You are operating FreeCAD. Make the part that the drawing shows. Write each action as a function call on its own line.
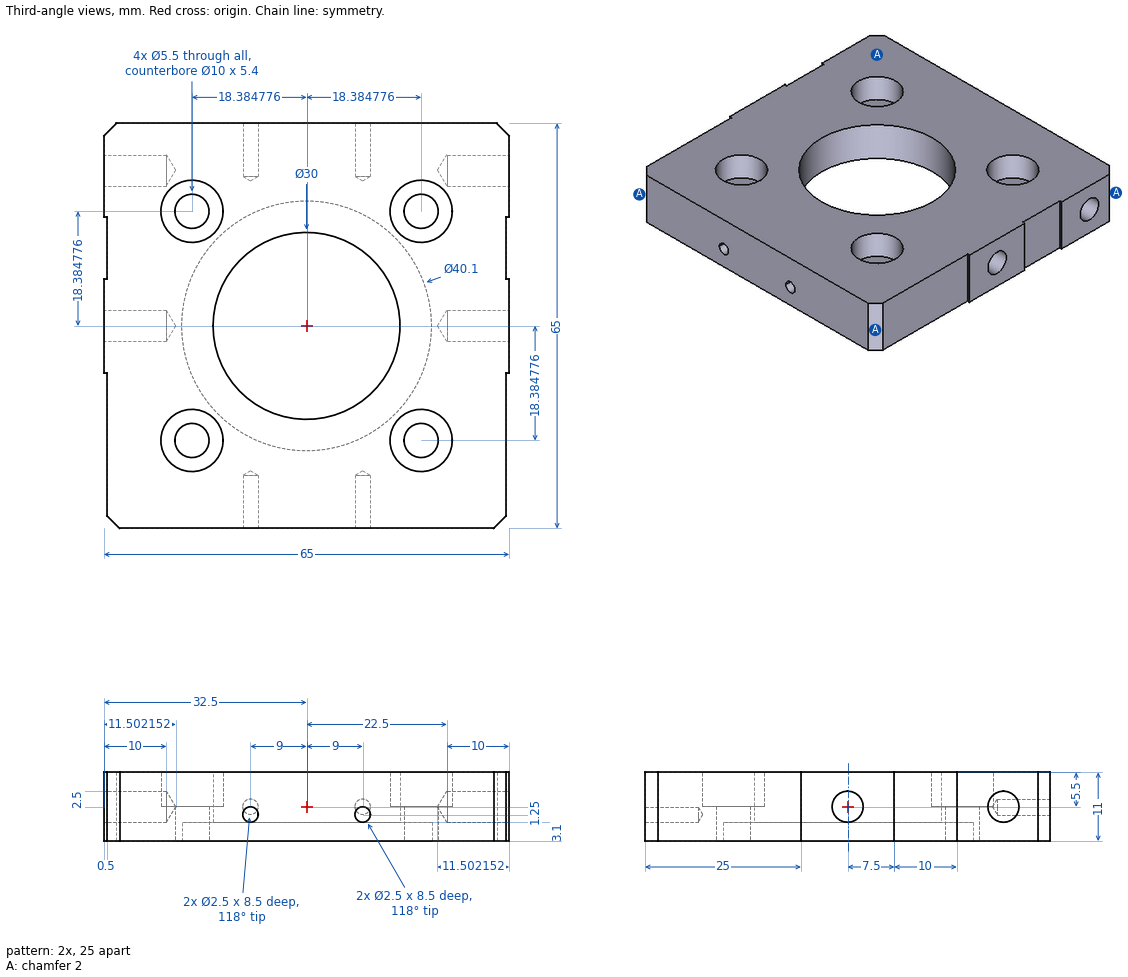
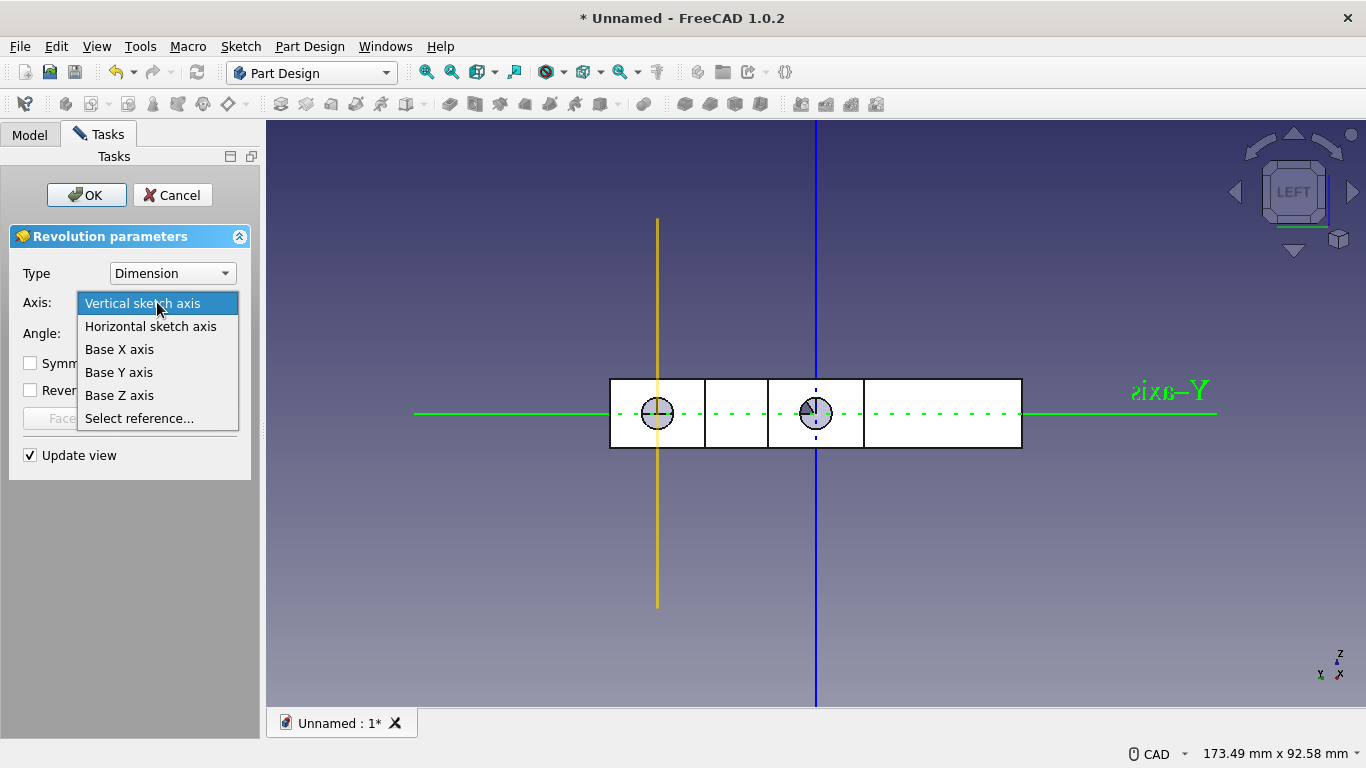
click(156, 326)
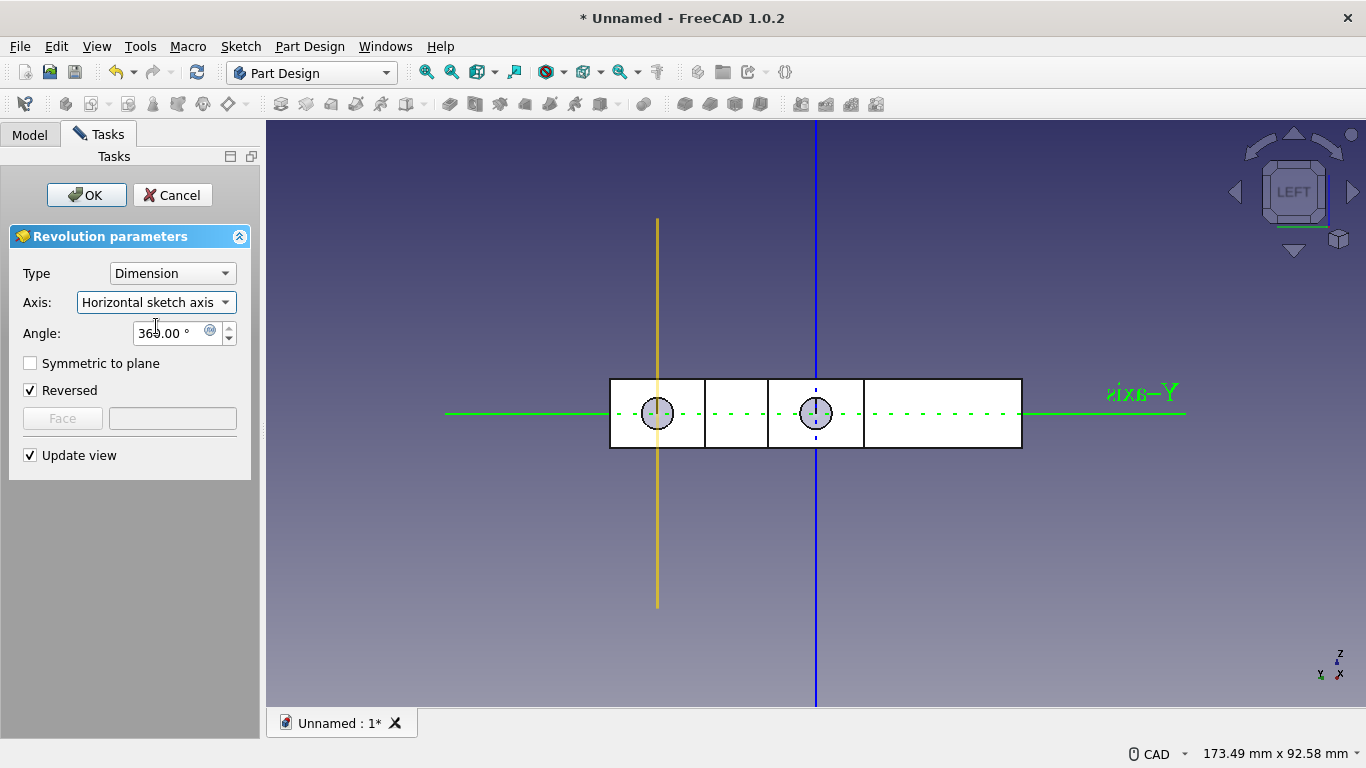
click(87, 195)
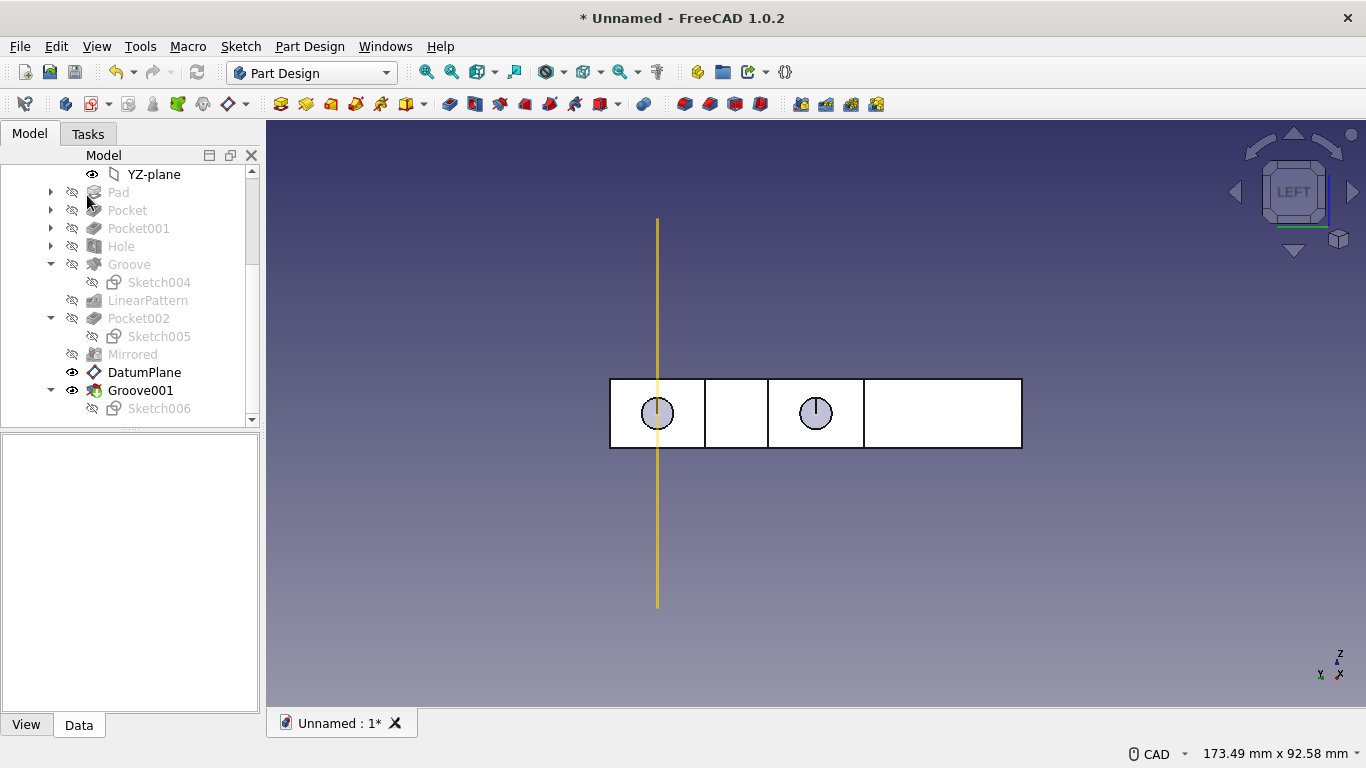
click(117, 372)
key(space)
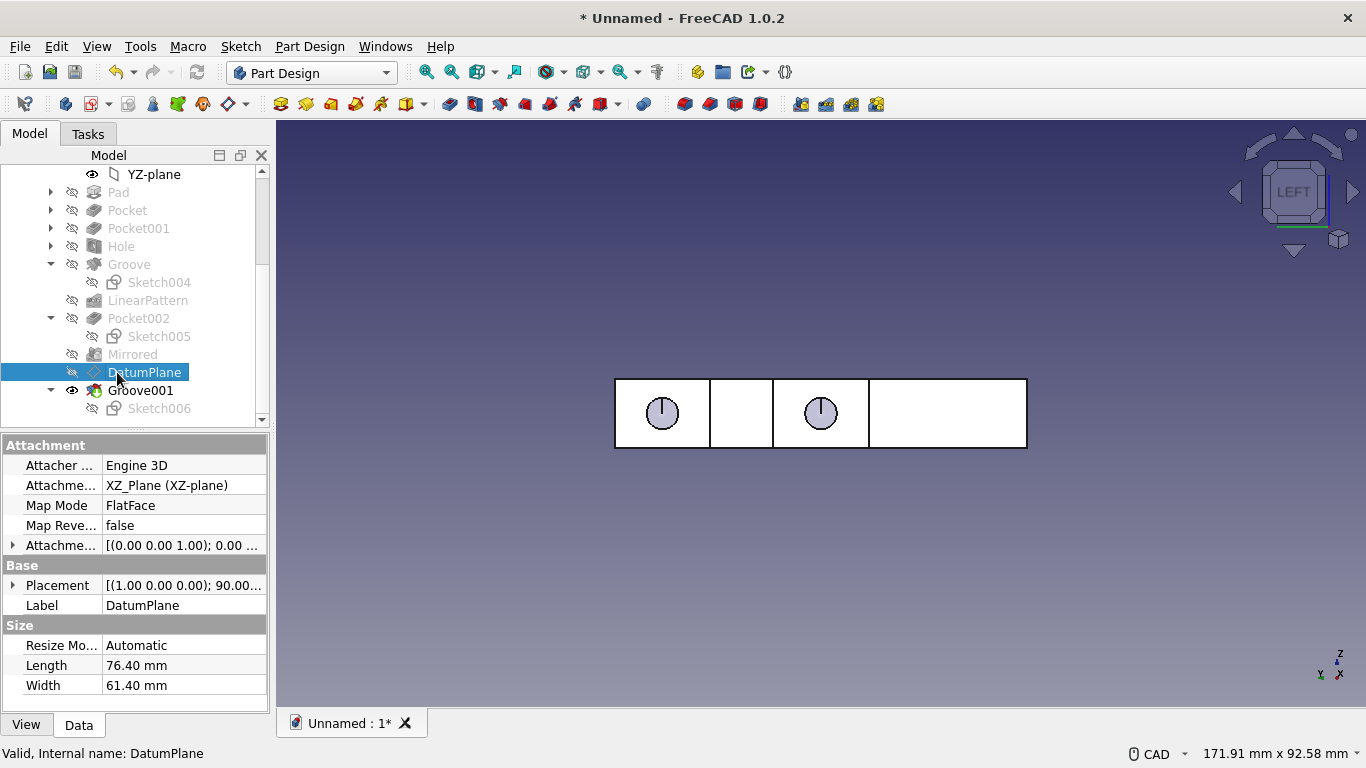
click(427, 72)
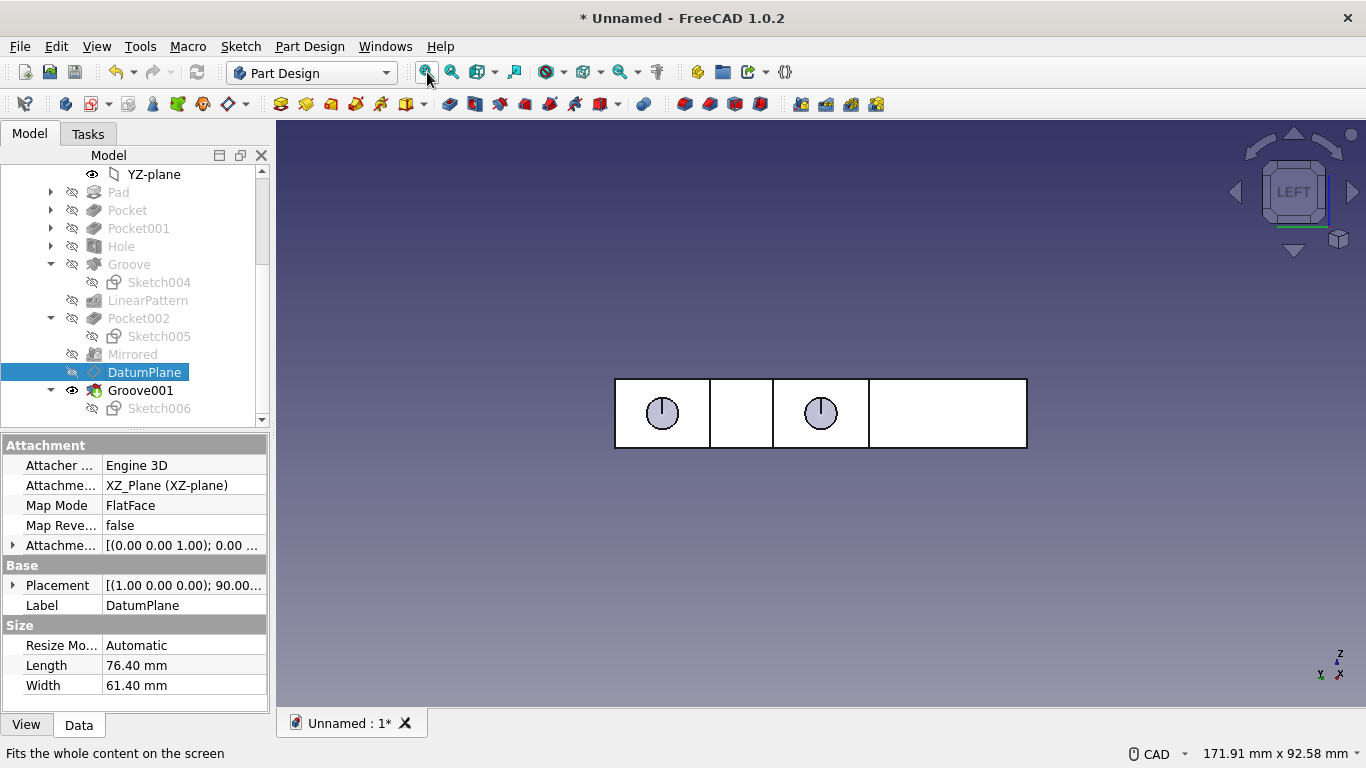
click(615, 412)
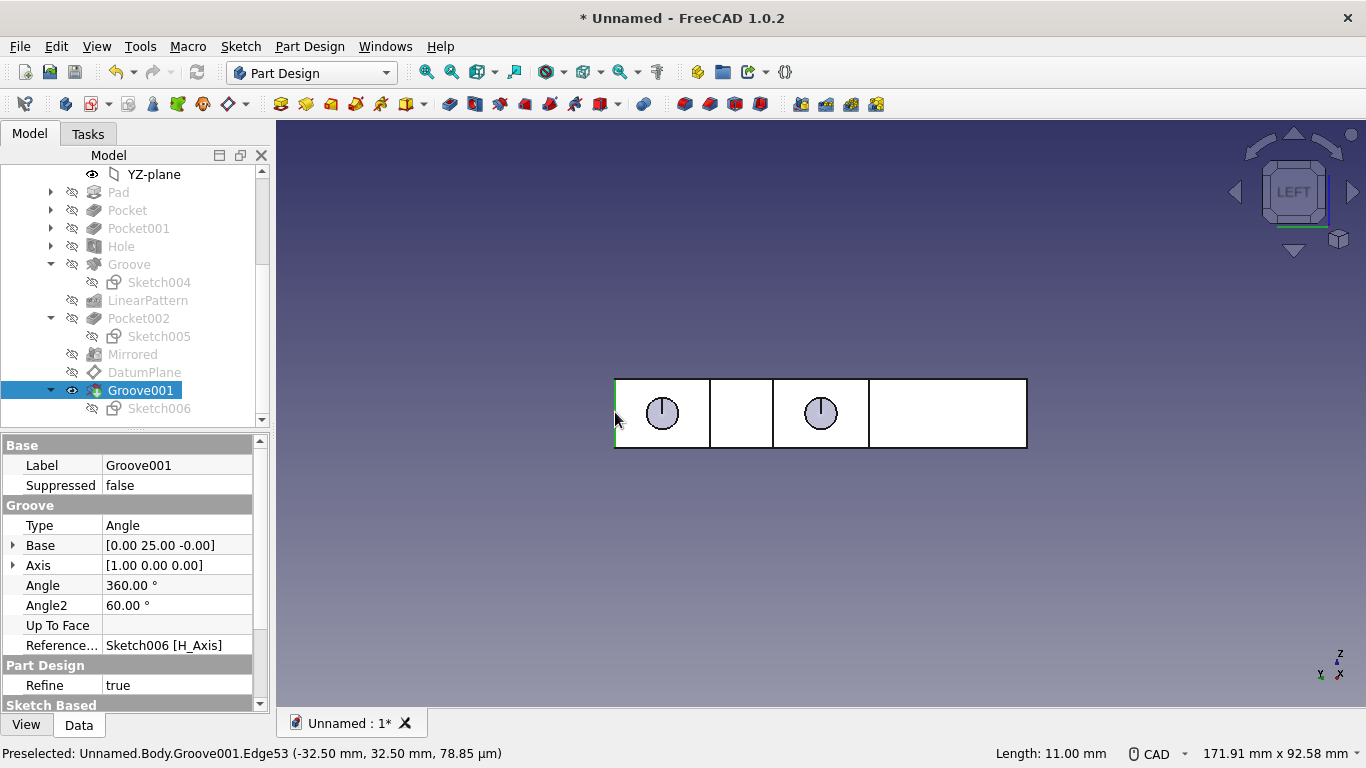
click(1027, 412, ctrl)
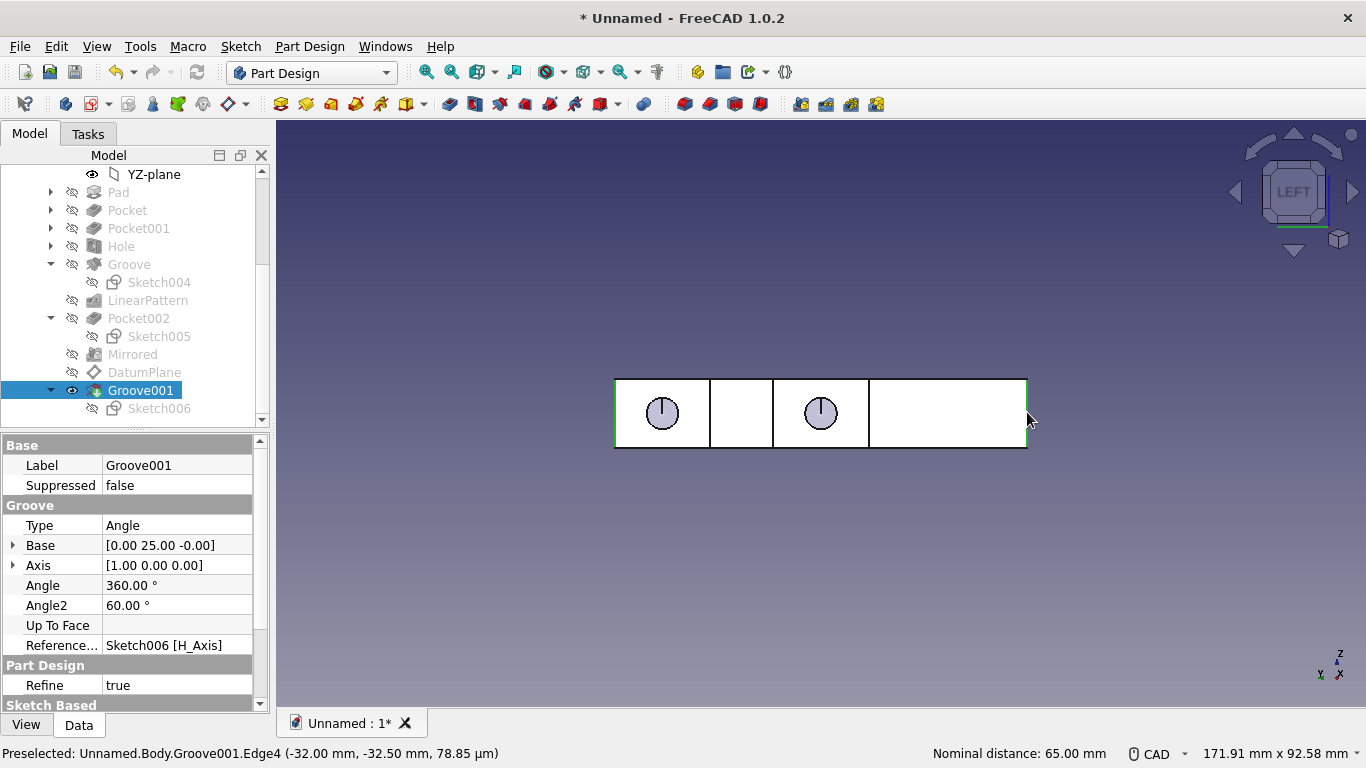
key(0)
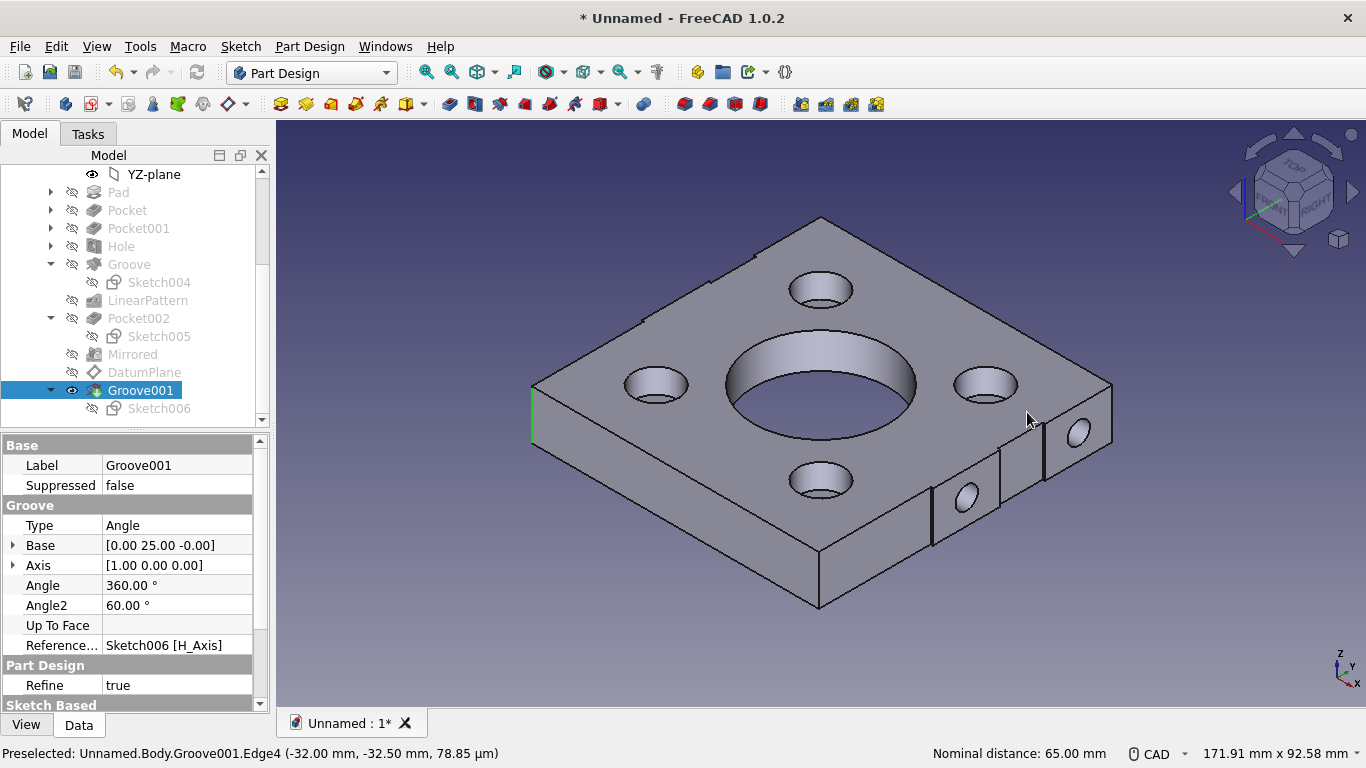
click(819, 579, ctrl)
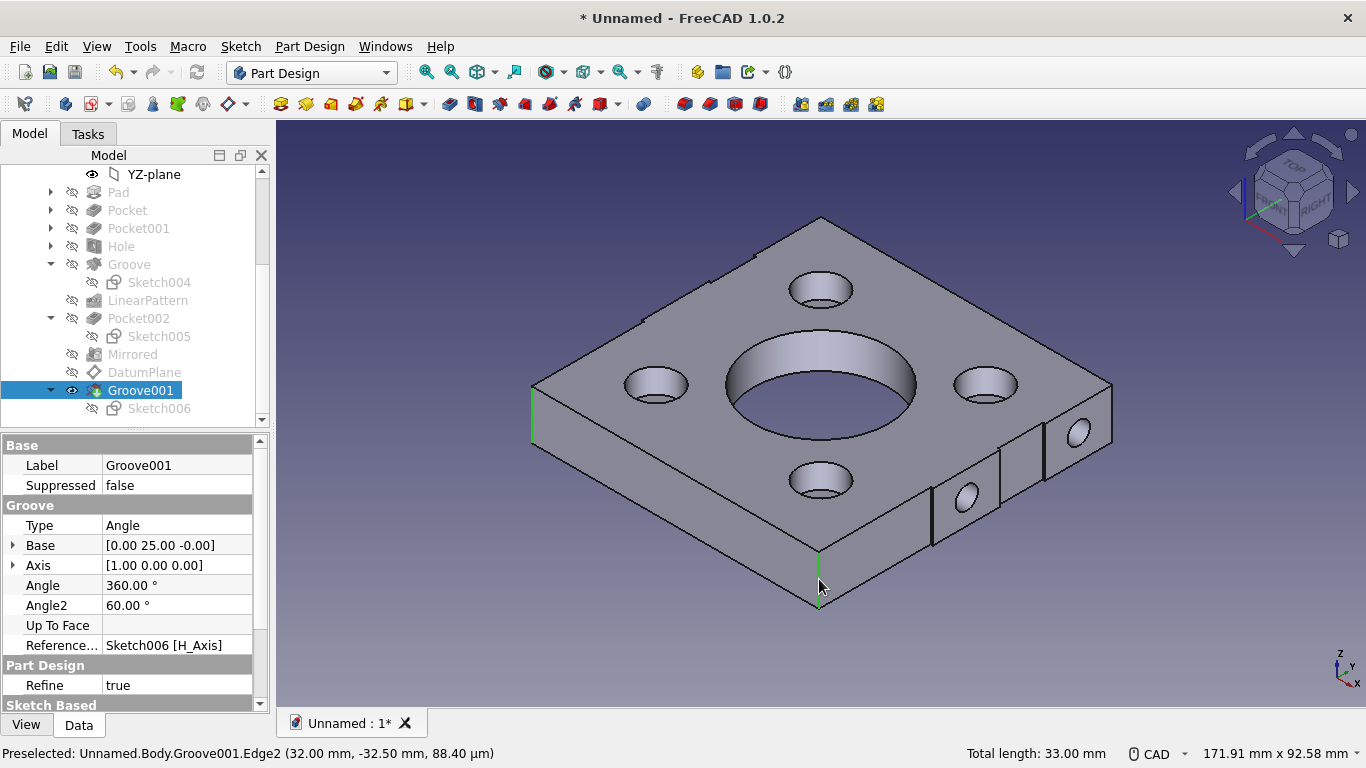
key(2)